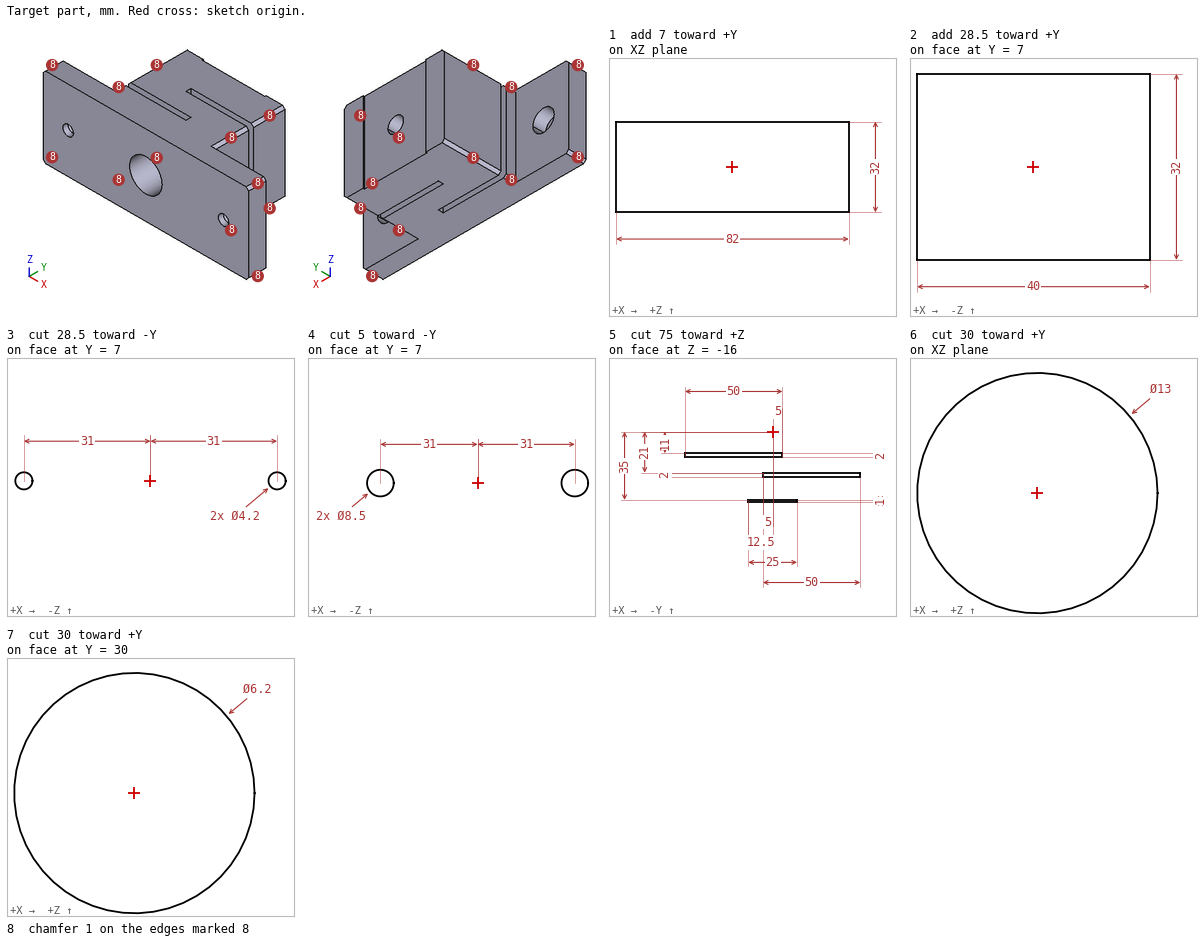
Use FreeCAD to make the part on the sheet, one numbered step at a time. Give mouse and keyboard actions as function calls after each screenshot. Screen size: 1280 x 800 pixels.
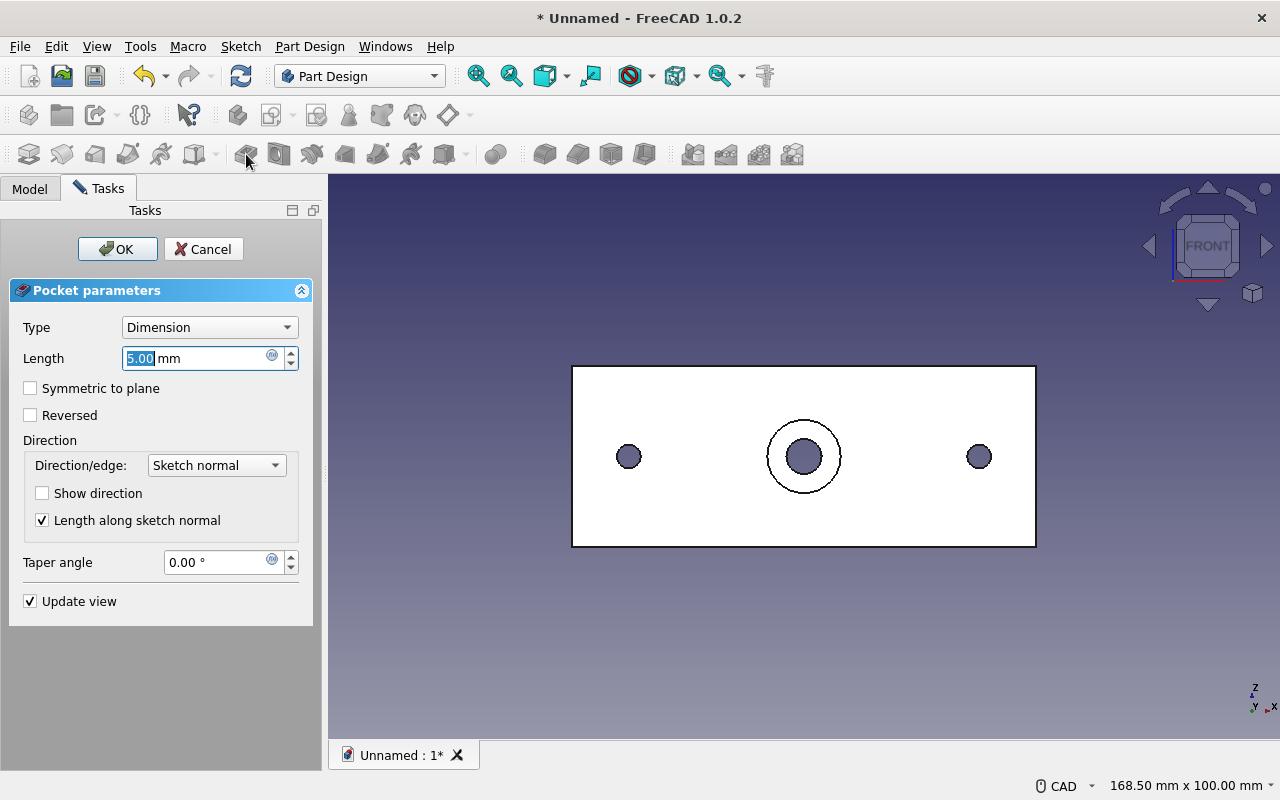
text(30)
key(Tab)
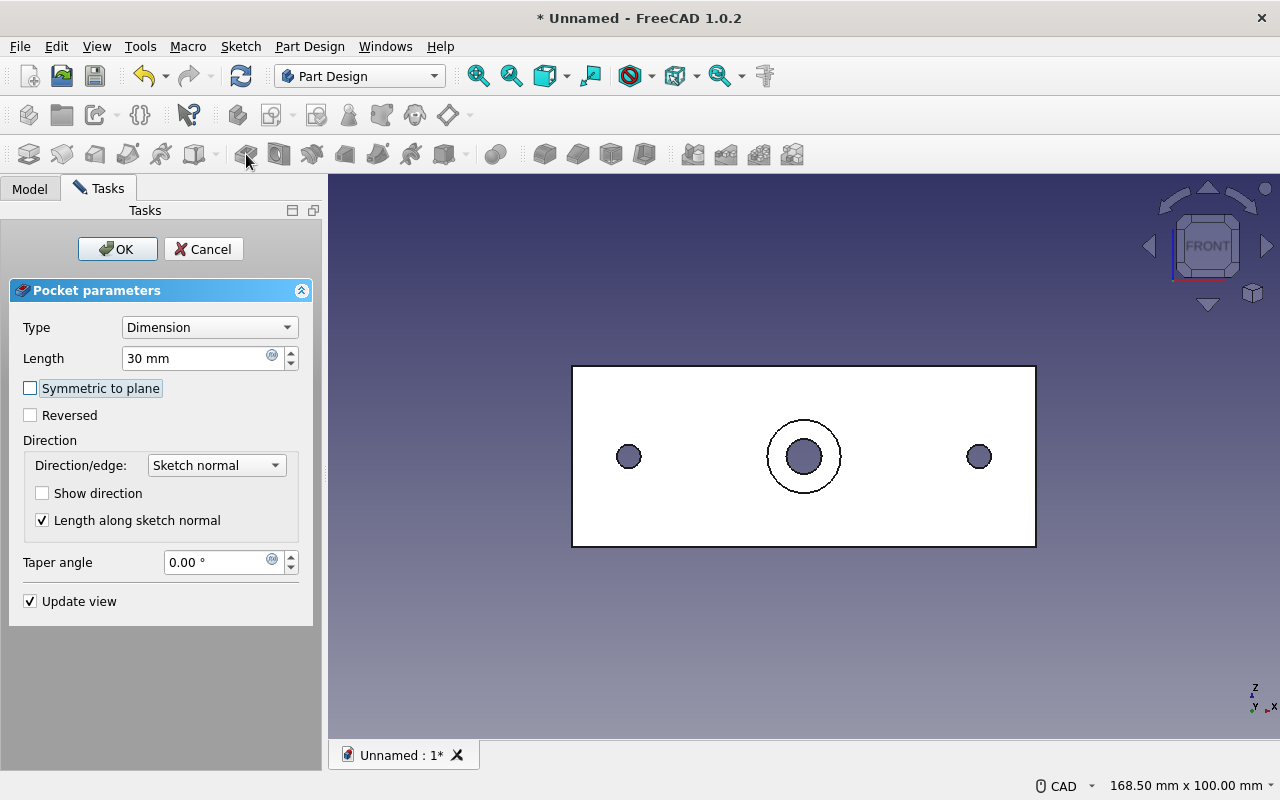
click(118, 249)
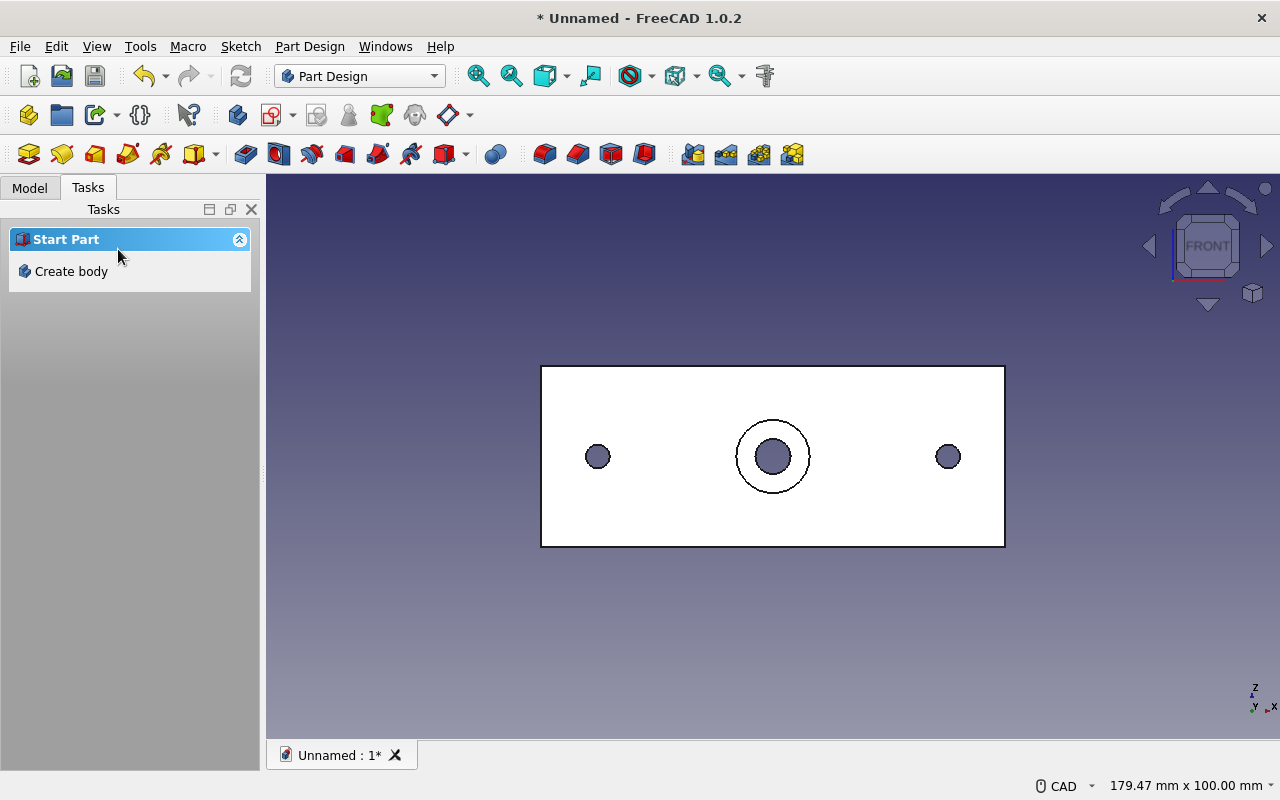
key(0)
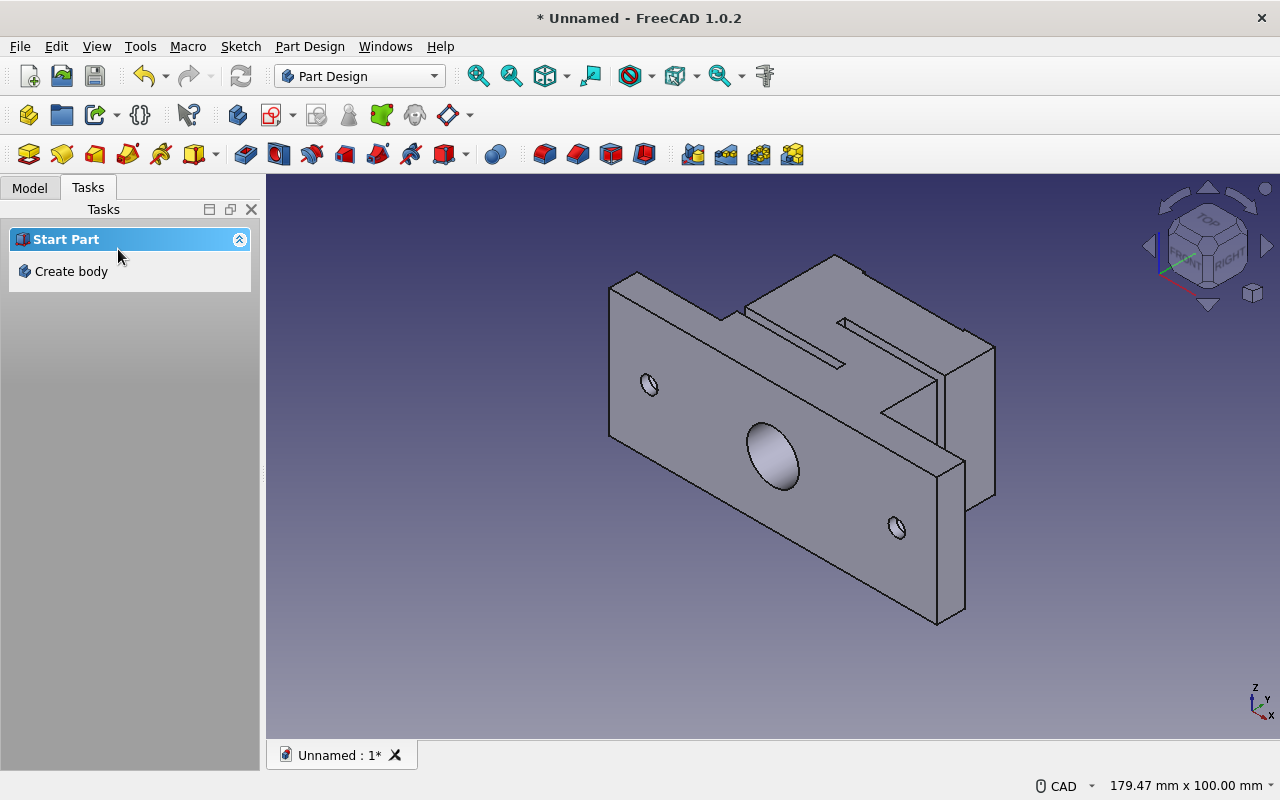
click(970, 360)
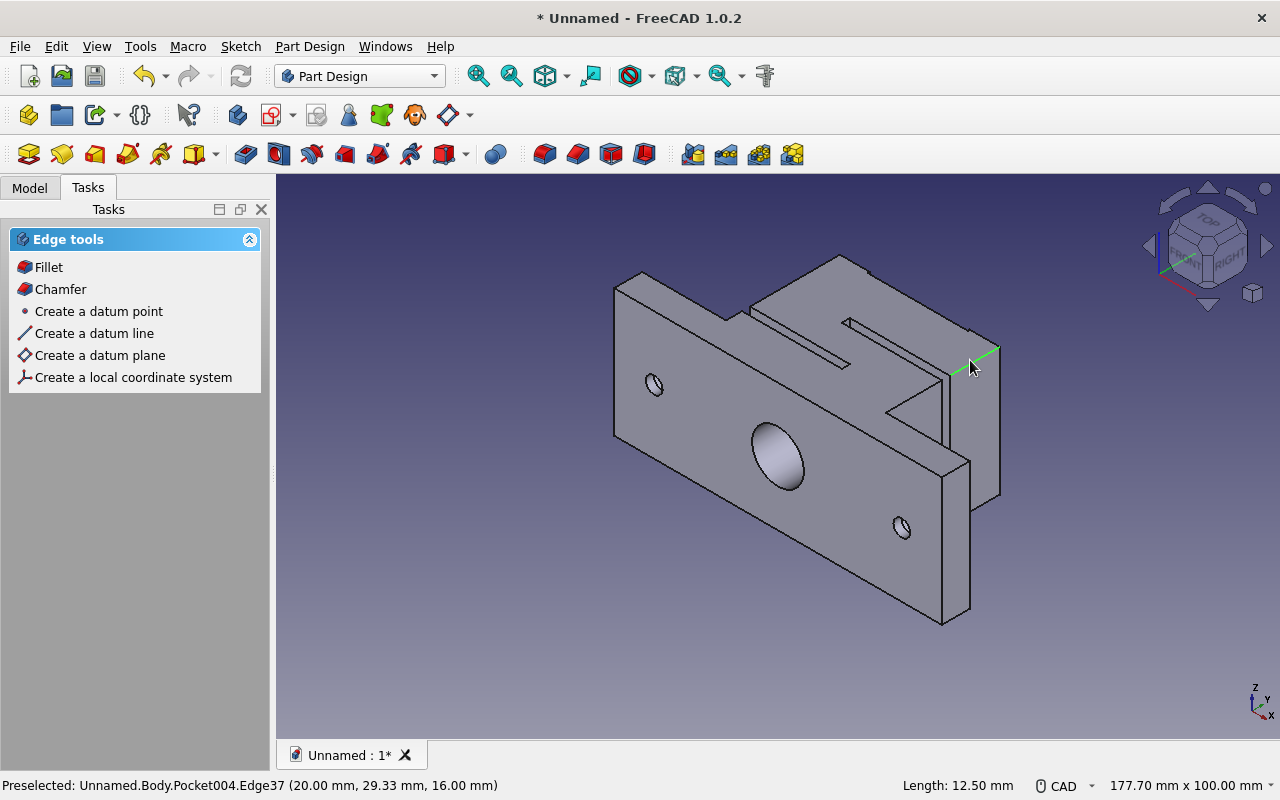
click(914, 396, ctrl)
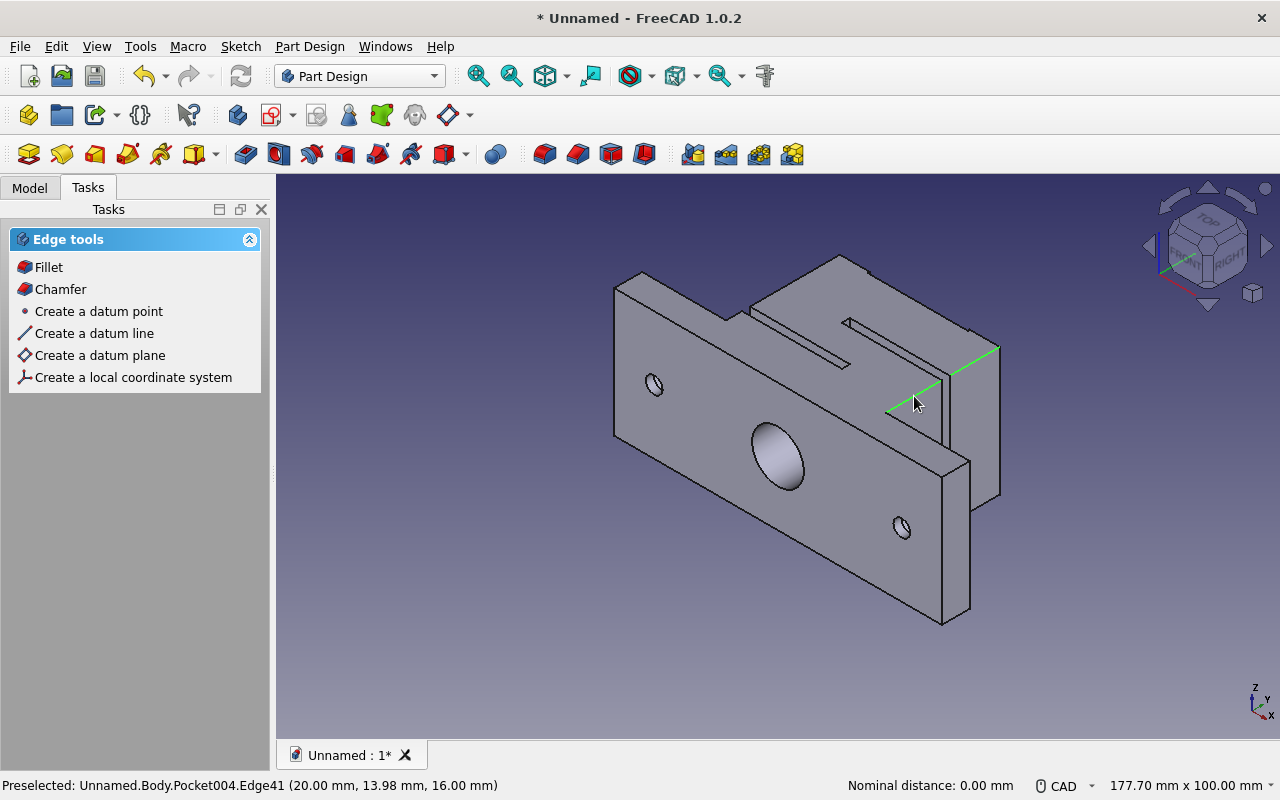
click(956, 468, ctrl)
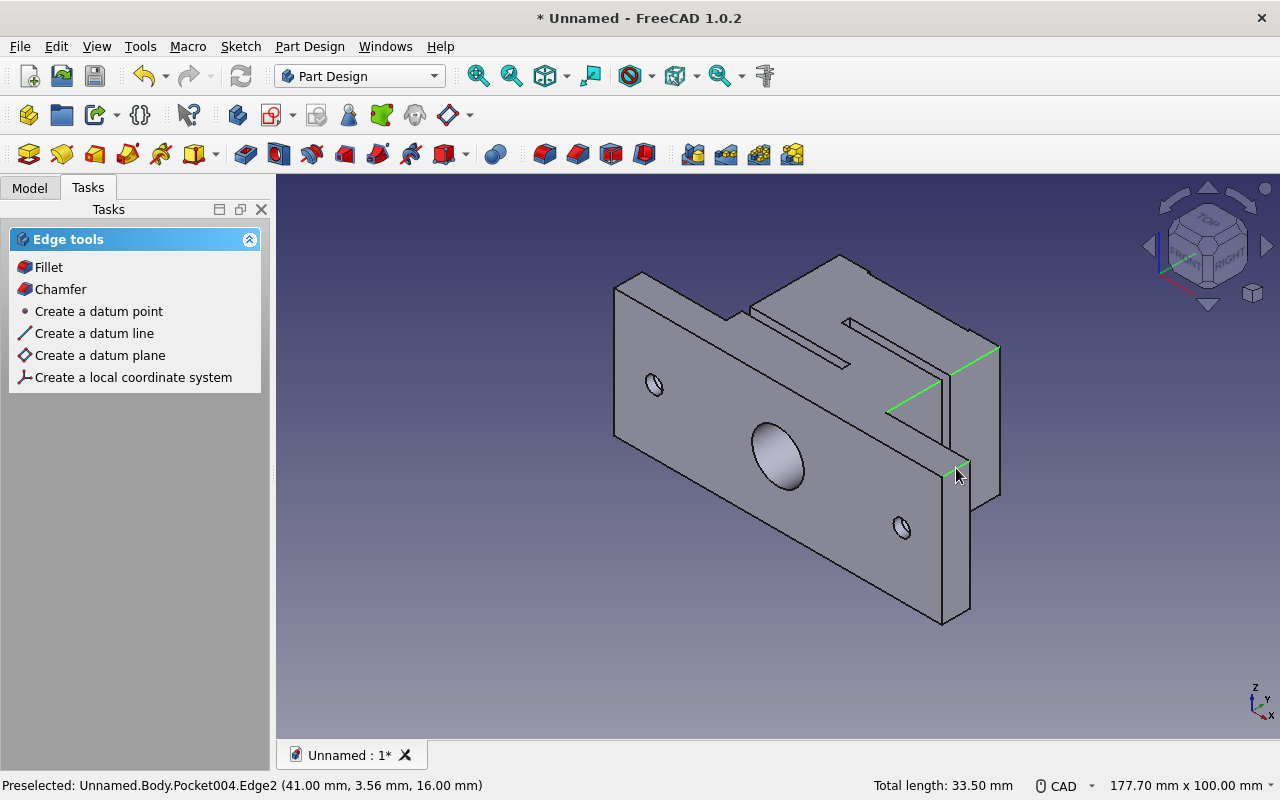
key(2)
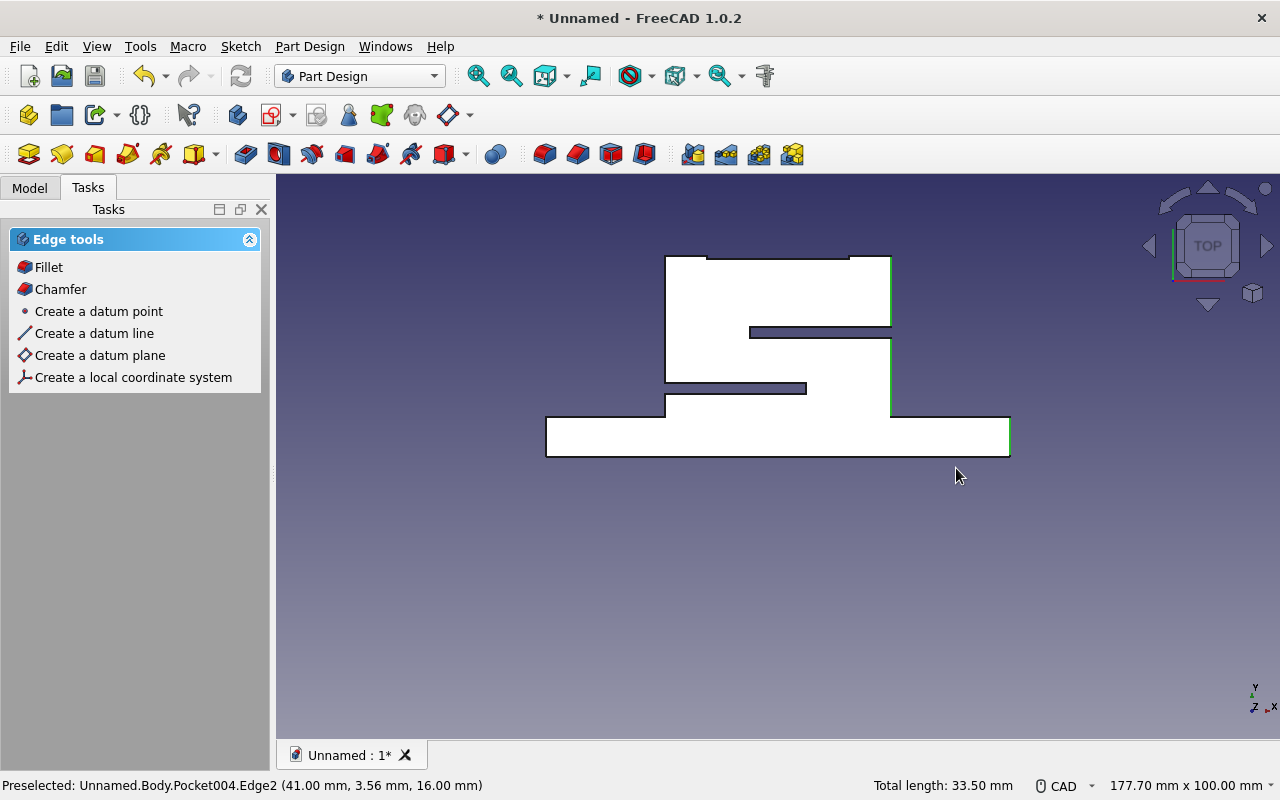
click(665, 318, ctrl)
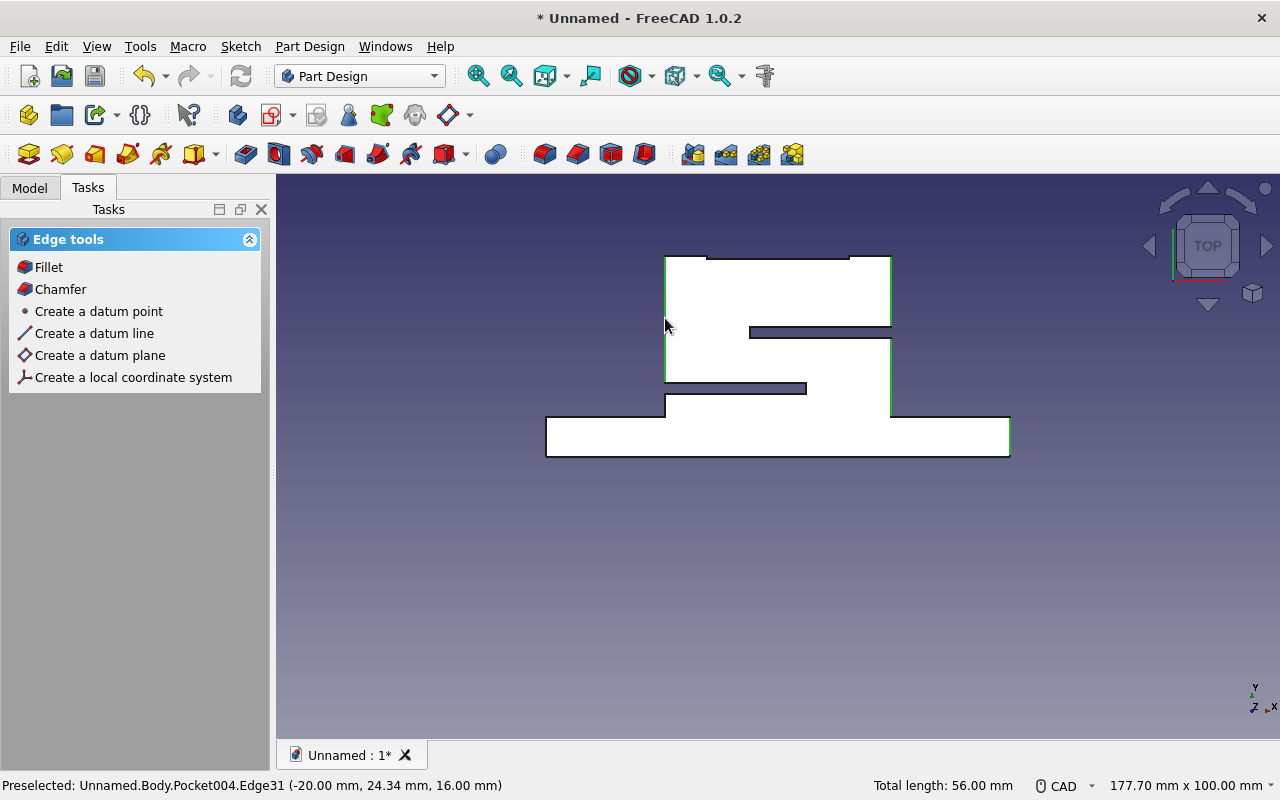
click(665, 405, ctrl)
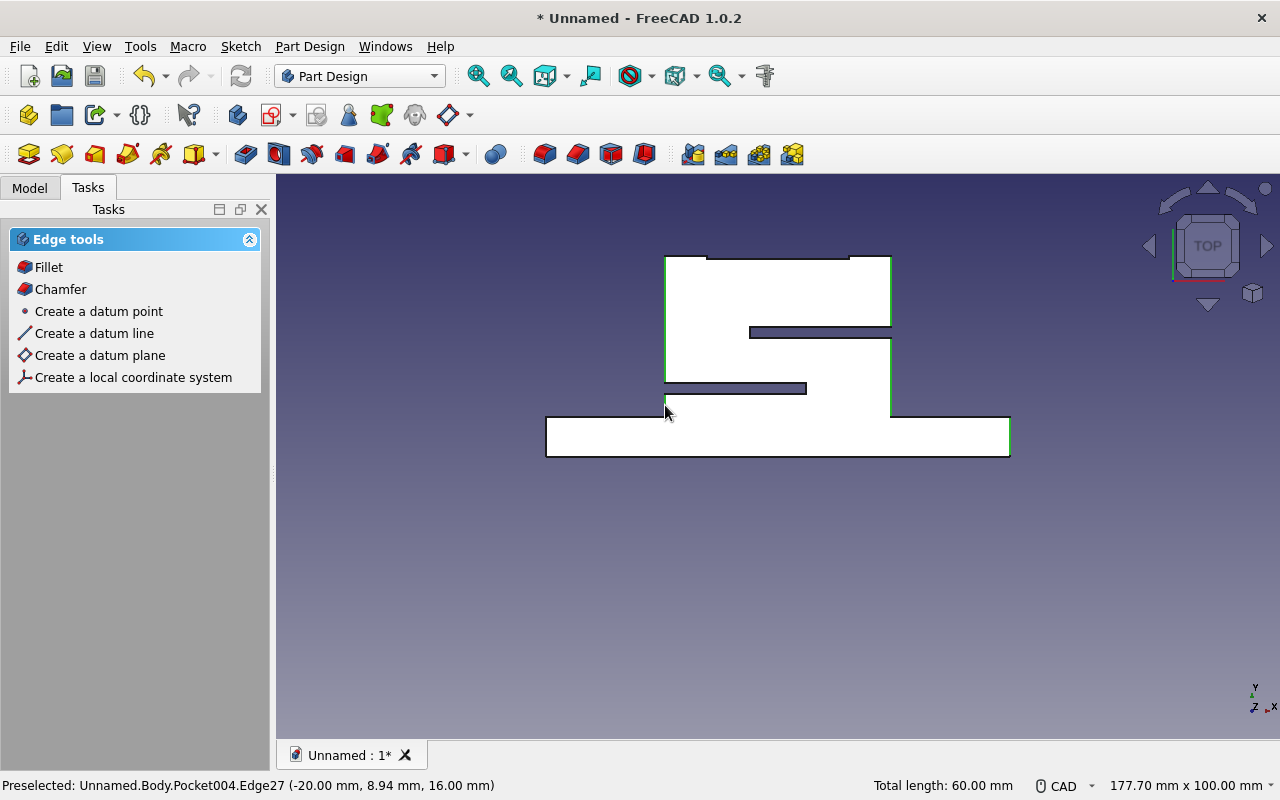
click(546, 436, ctrl)